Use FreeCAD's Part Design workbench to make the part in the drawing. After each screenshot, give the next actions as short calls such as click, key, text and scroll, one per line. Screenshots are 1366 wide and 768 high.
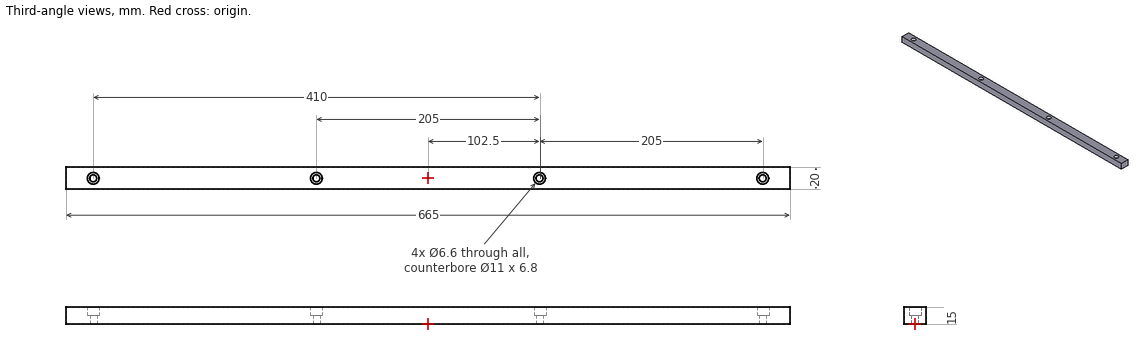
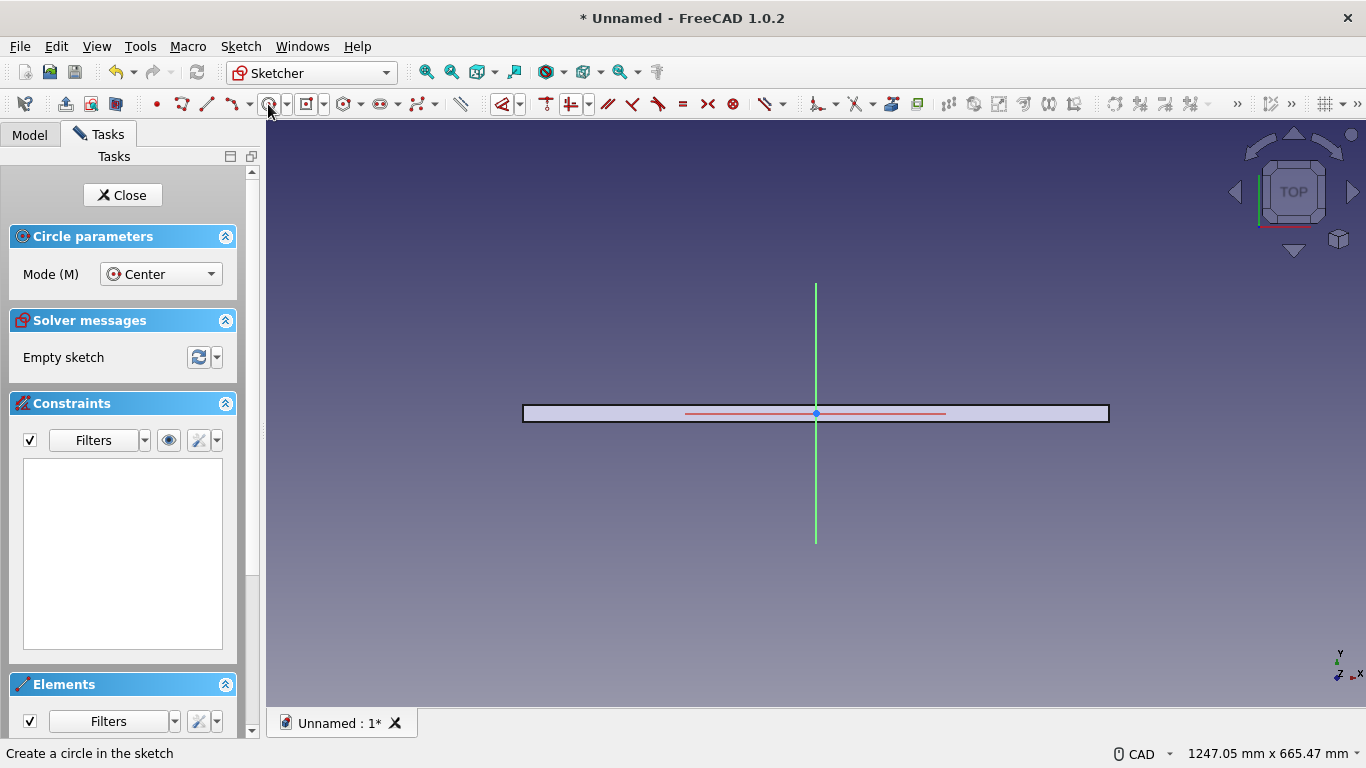
scroll(906, 414, up, 11)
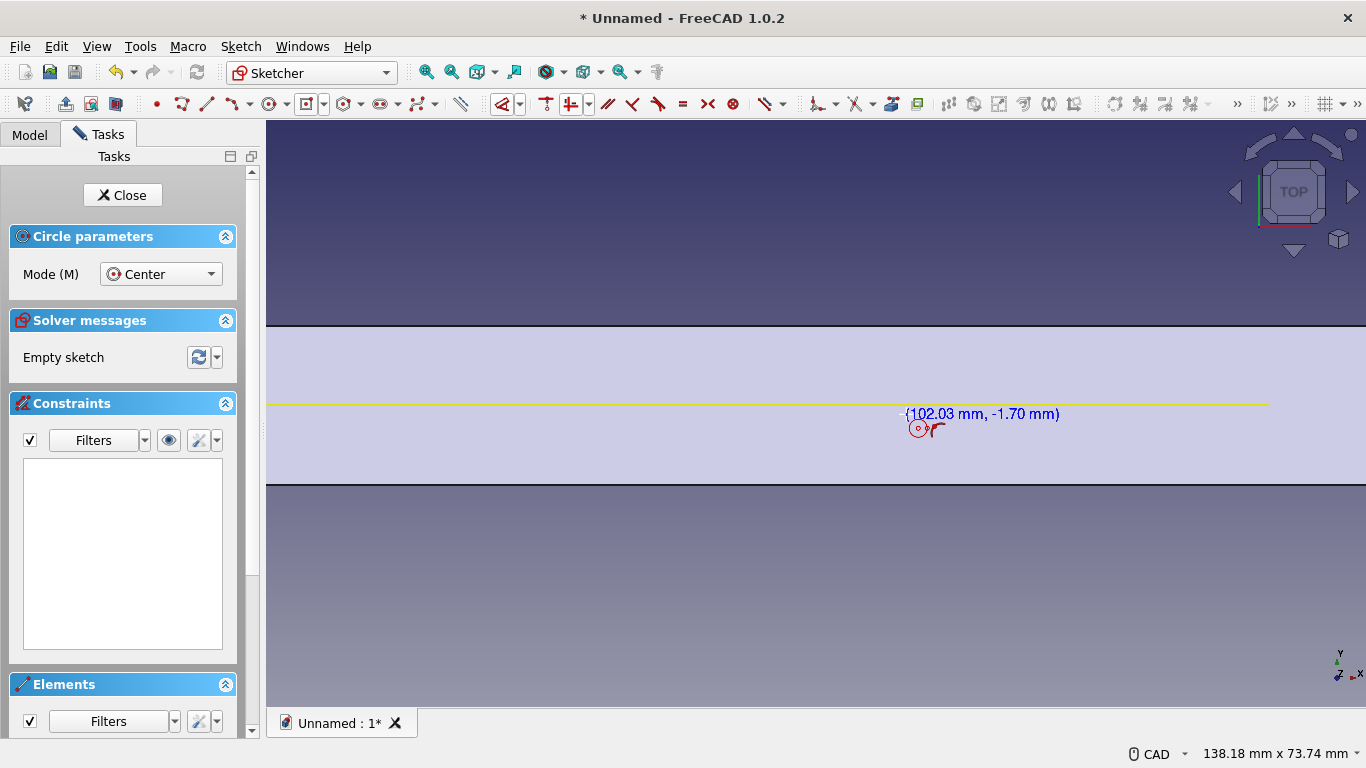
scroll(851, 415, down, 10)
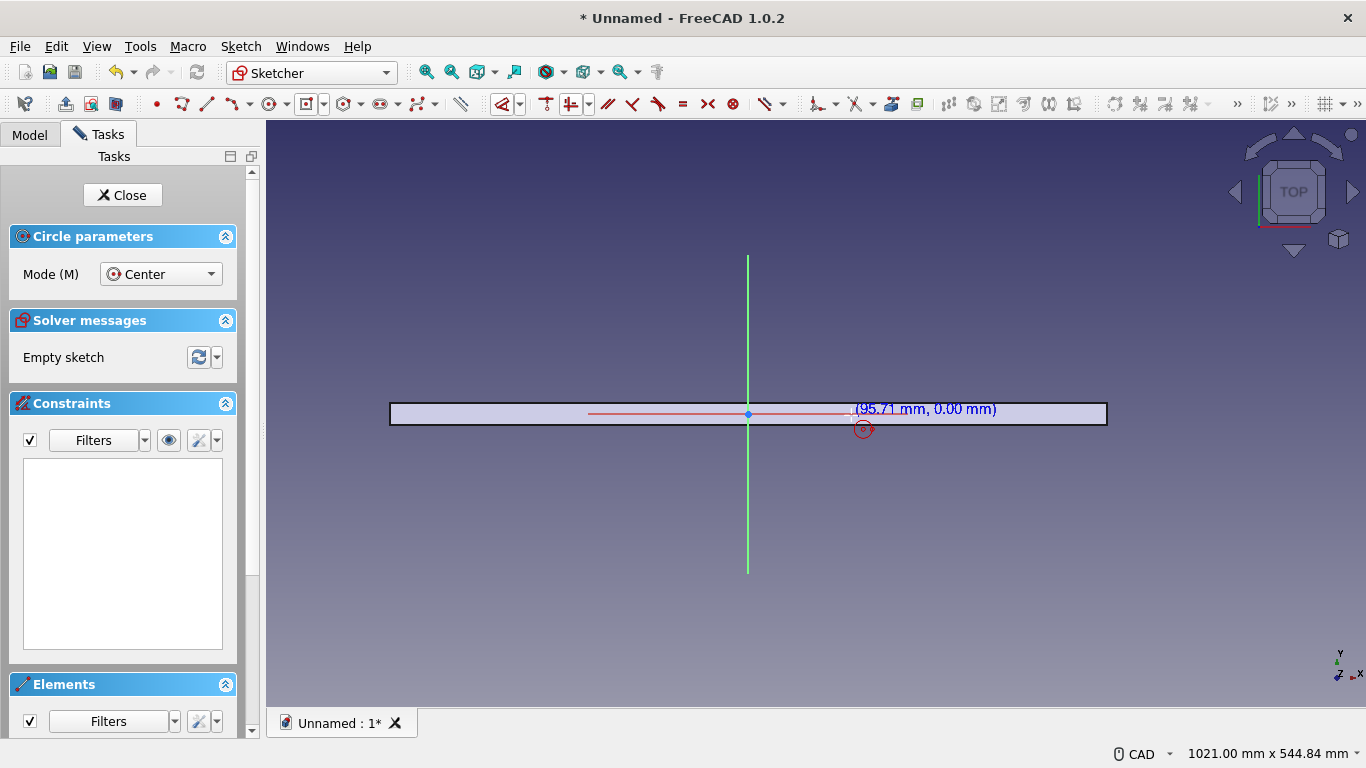
click(859, 414)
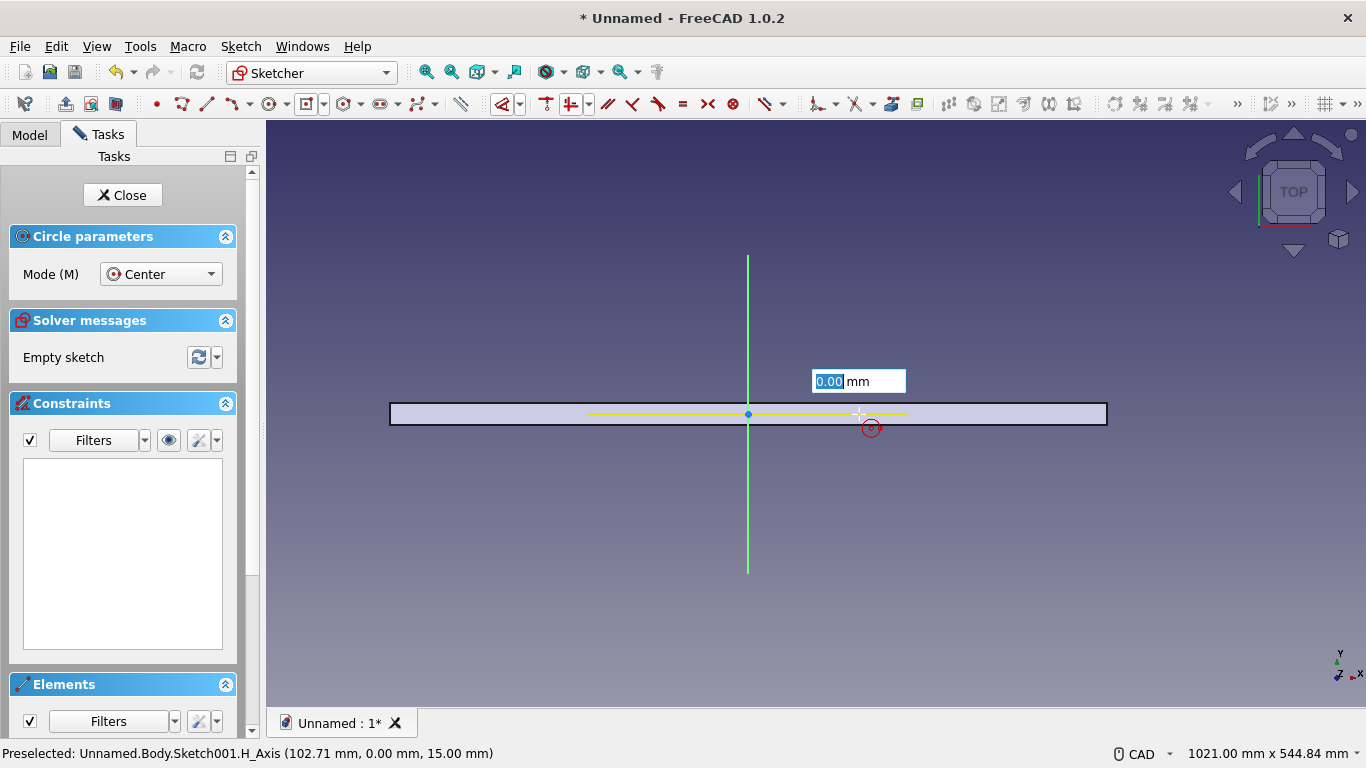
scroll(858, 417, up, 8)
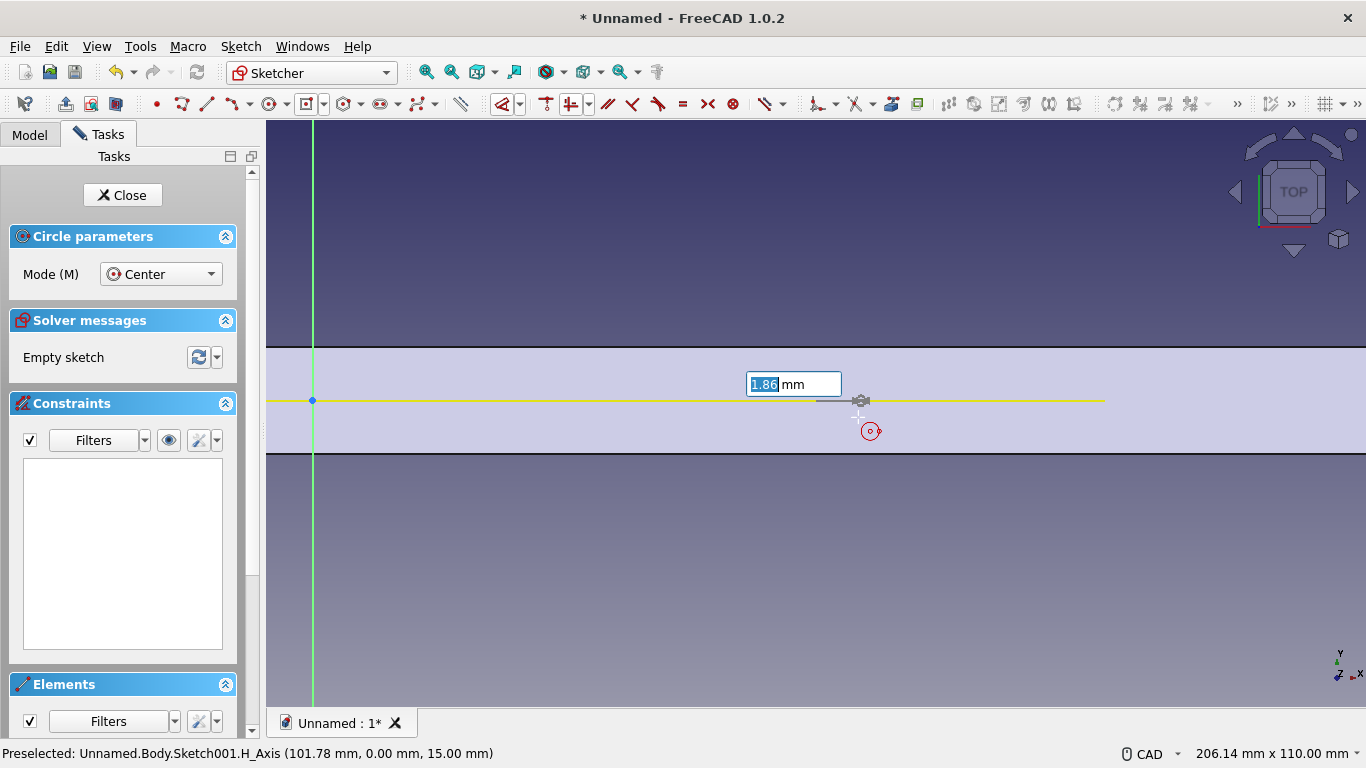
click(854, 417)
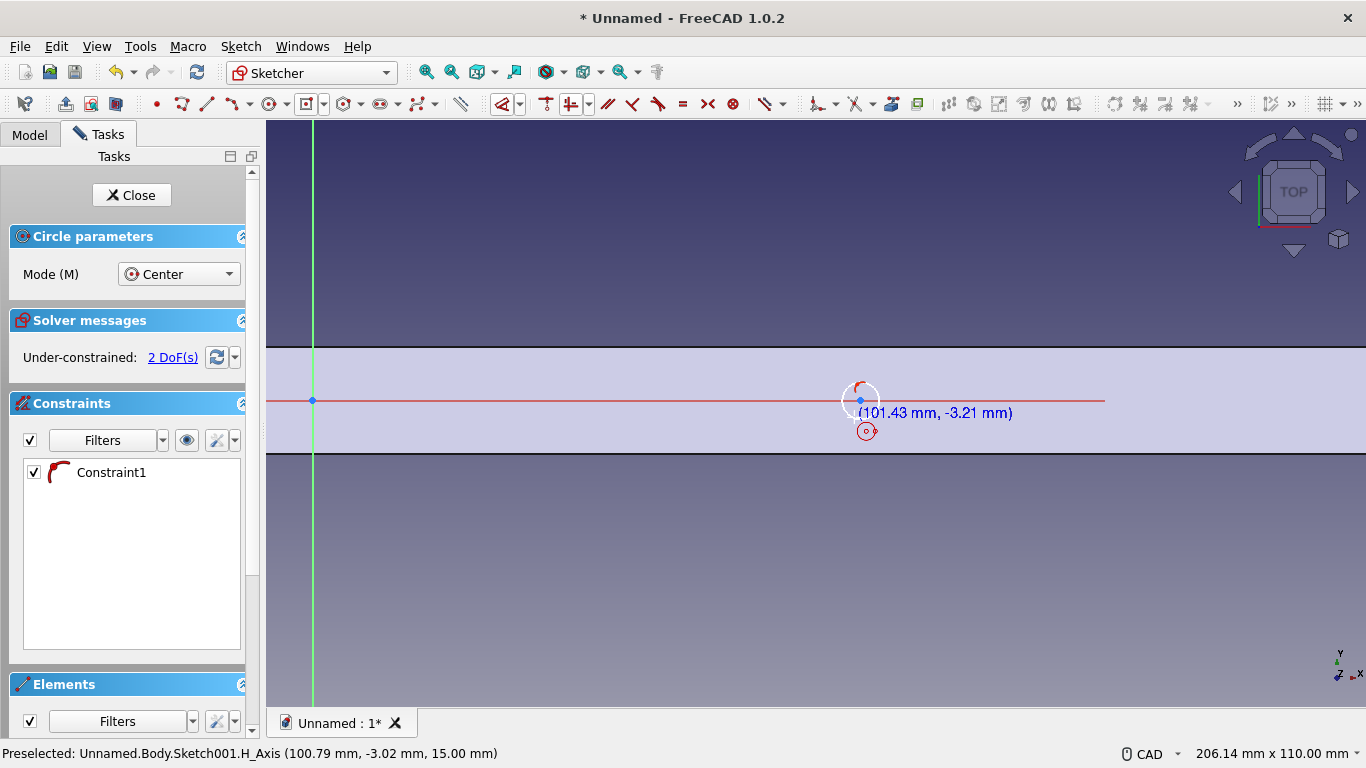
scroll(857, 417, down, 8)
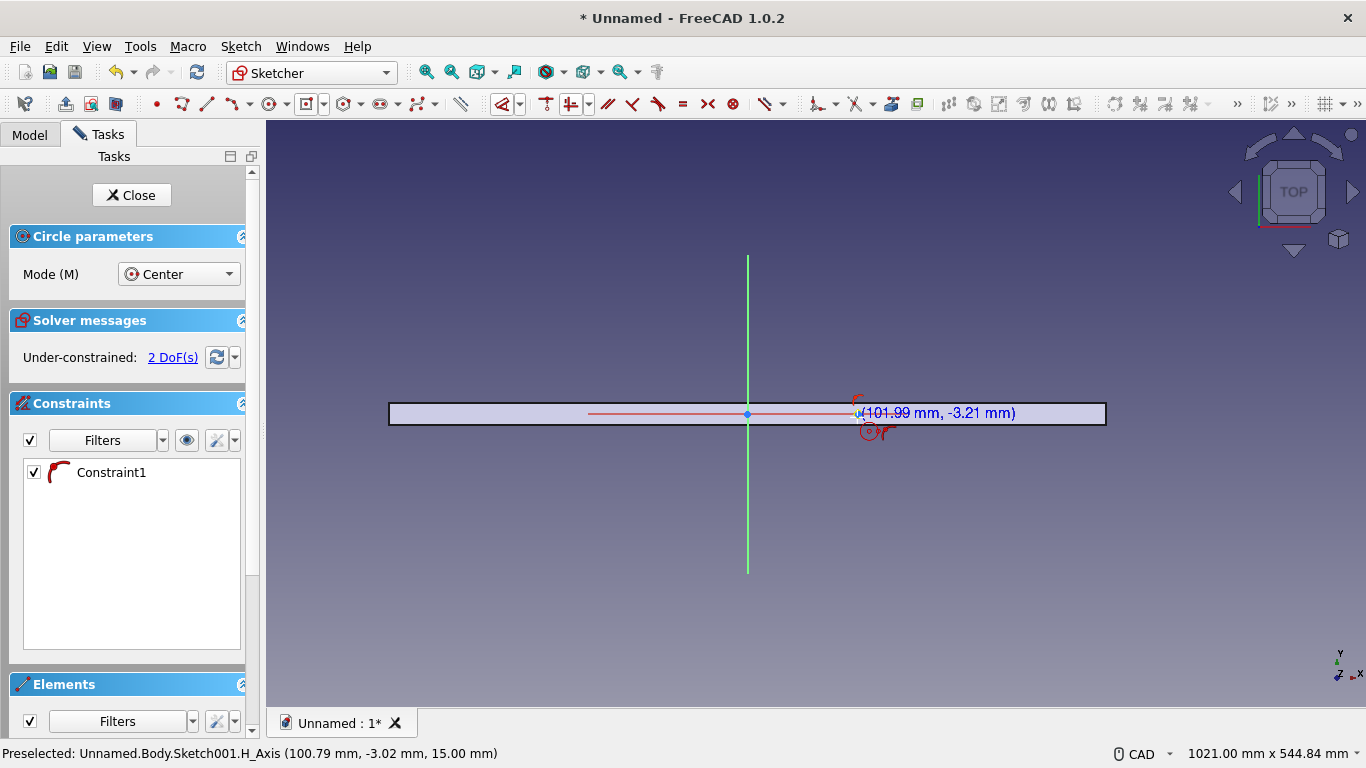
scroll(416, 414, up, 10)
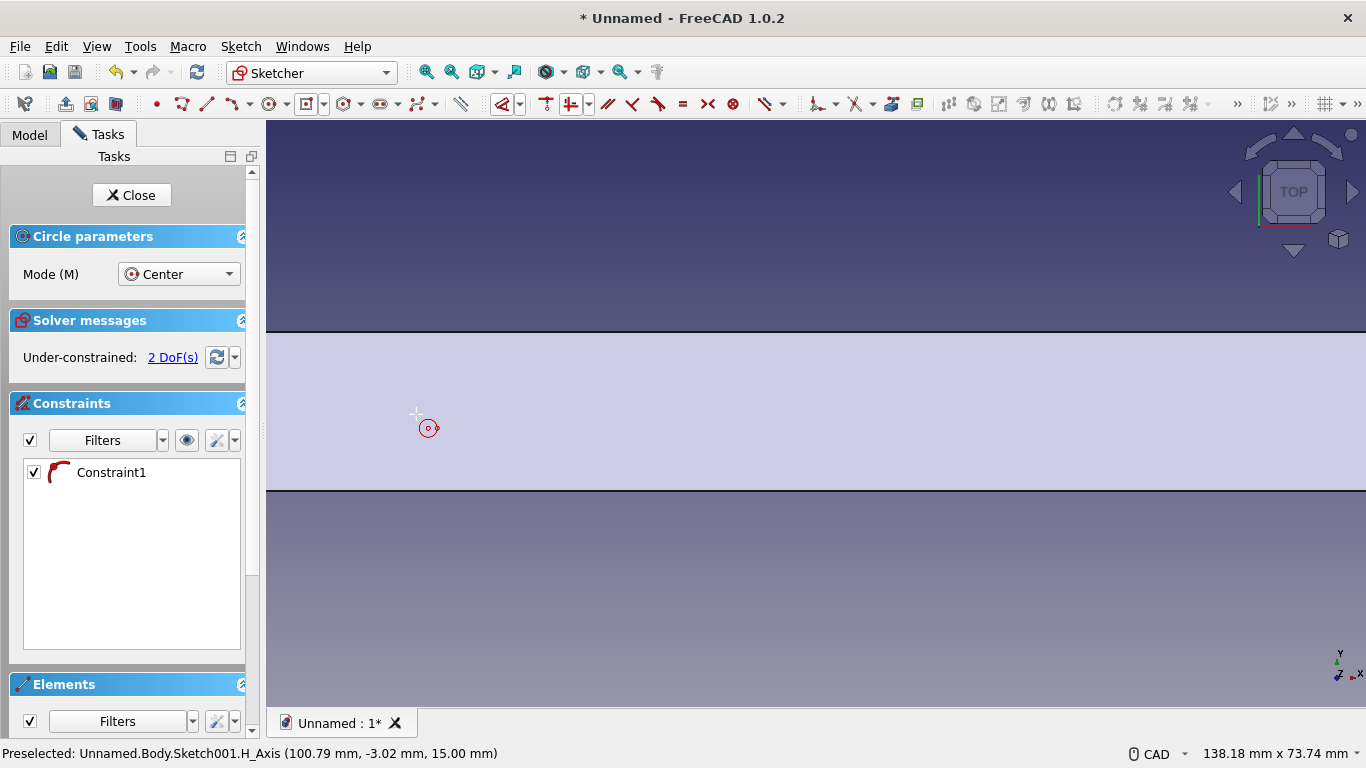
scroll(416, 414, down, 10)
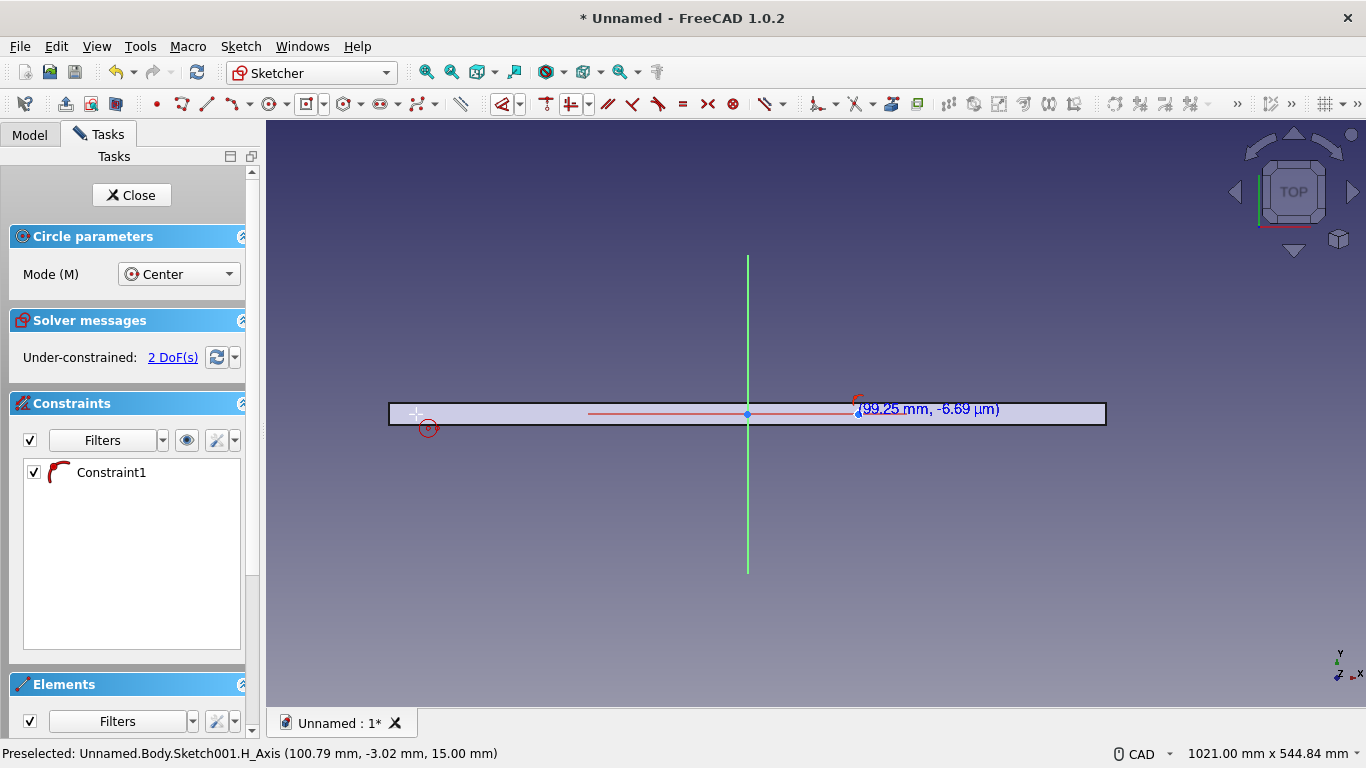
click(416, 414)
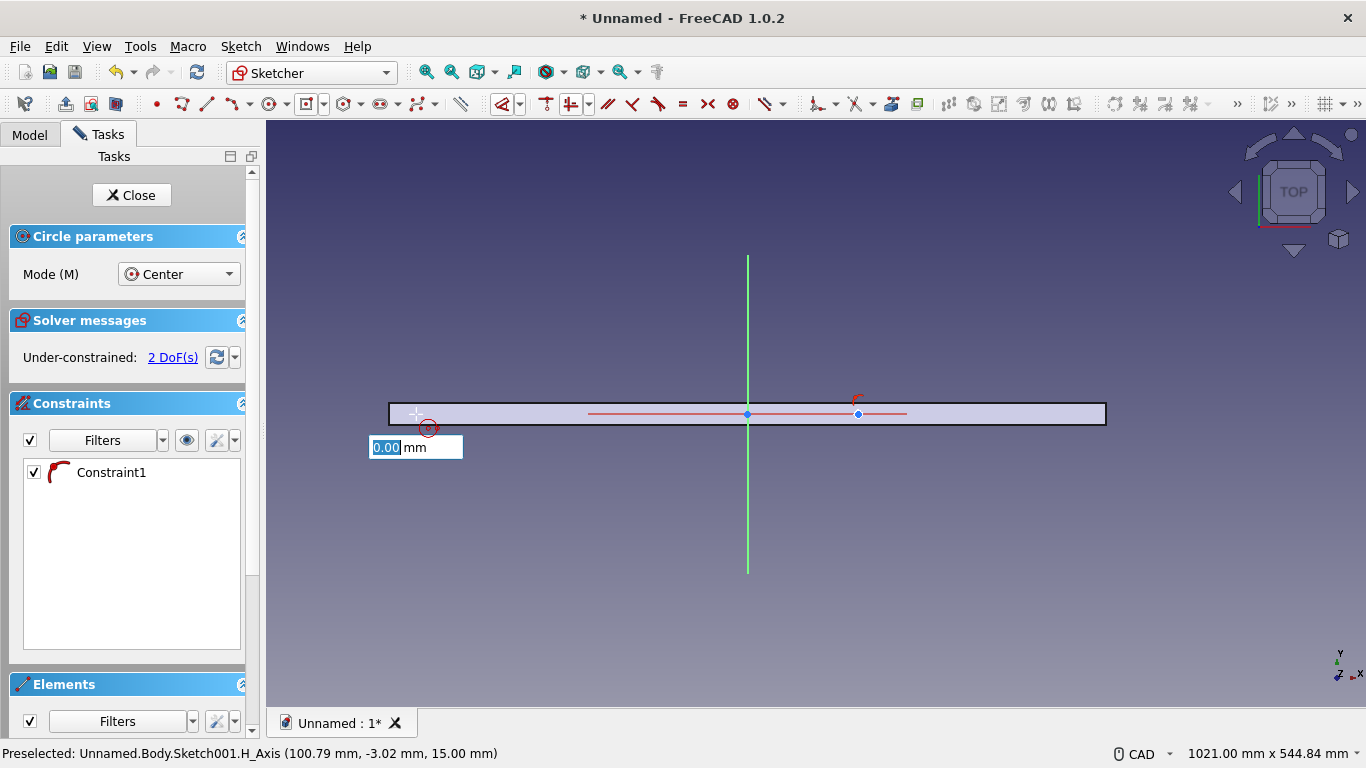
scroll(415, 417, up, 8)